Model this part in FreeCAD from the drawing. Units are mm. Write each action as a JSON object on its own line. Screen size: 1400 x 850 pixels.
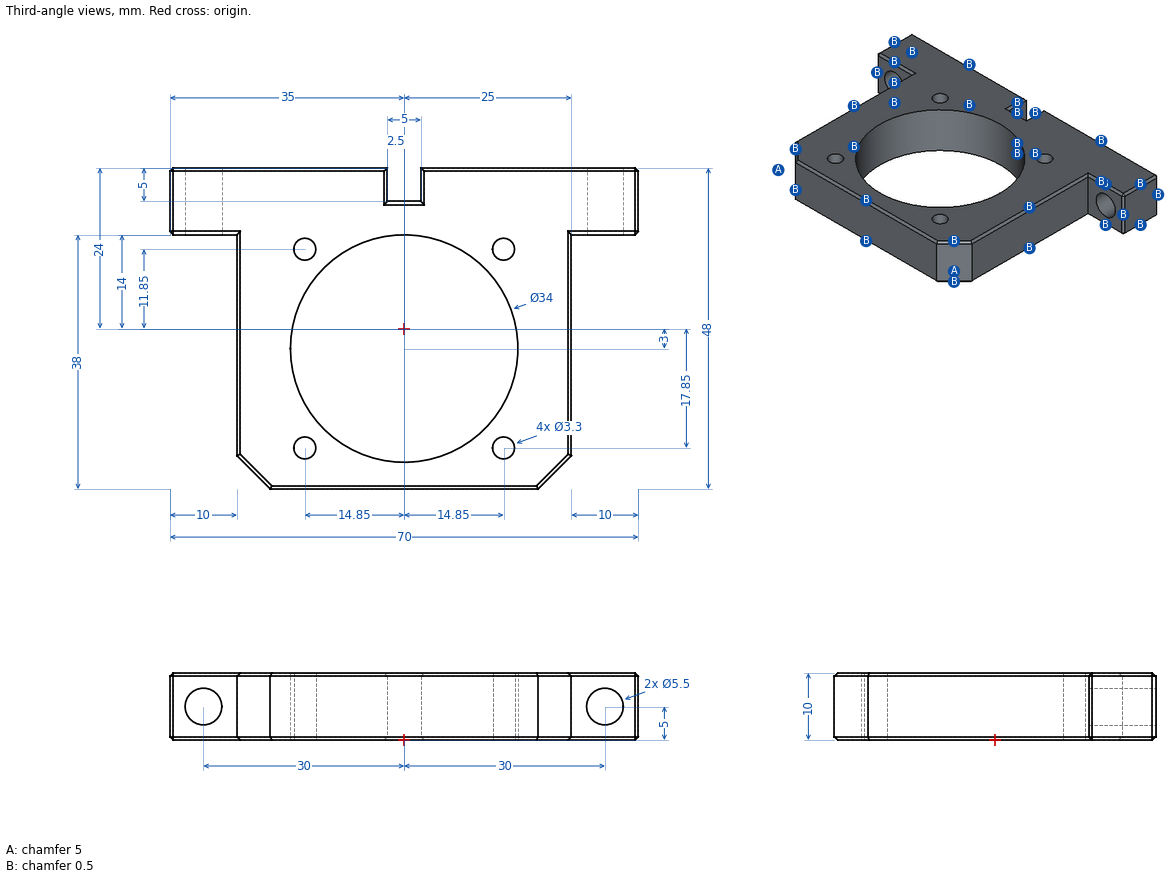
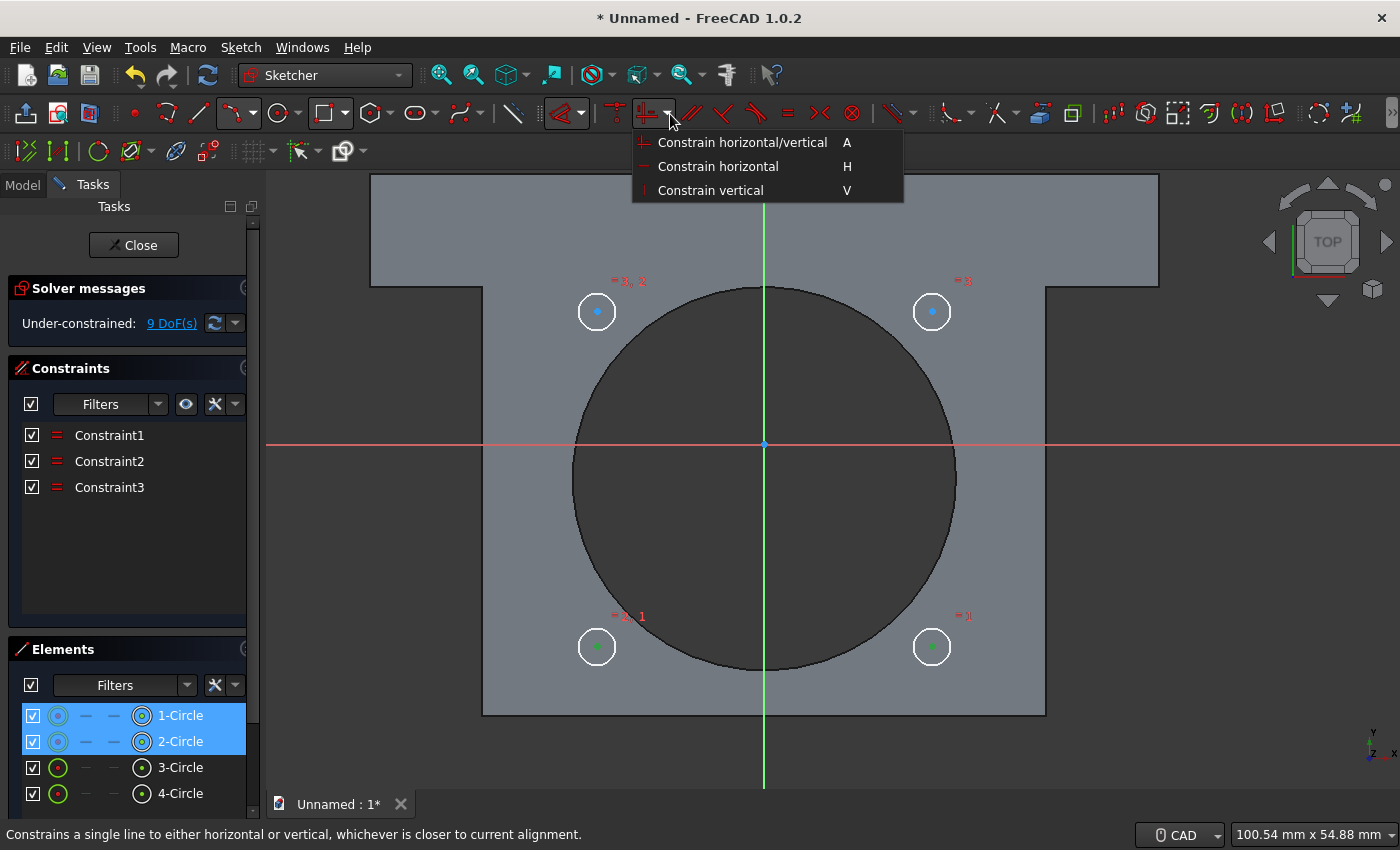
{"action": "left_click", "coordinate": [768, 166]}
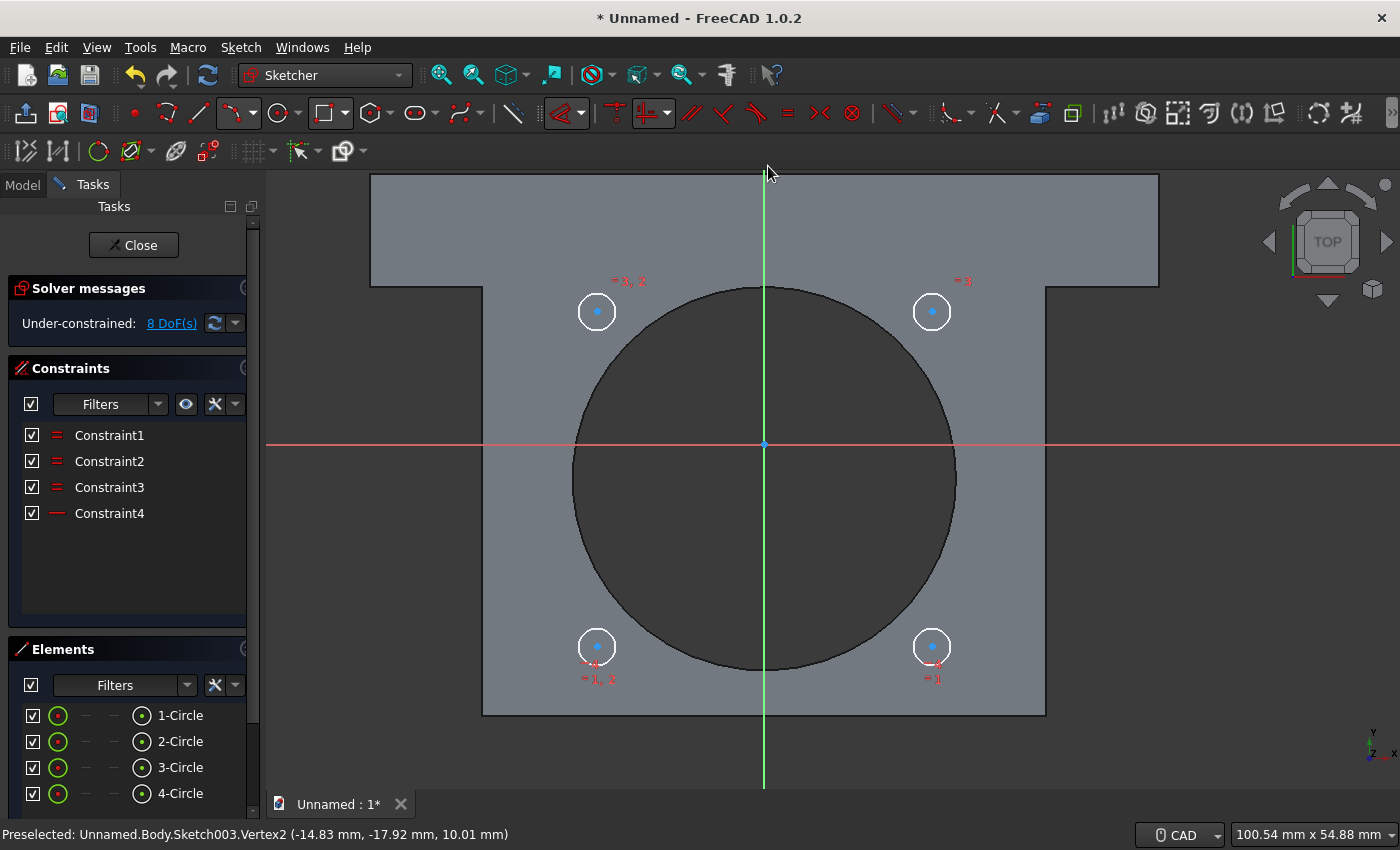
{"action": "left_click", "coordinate": [597, 647]}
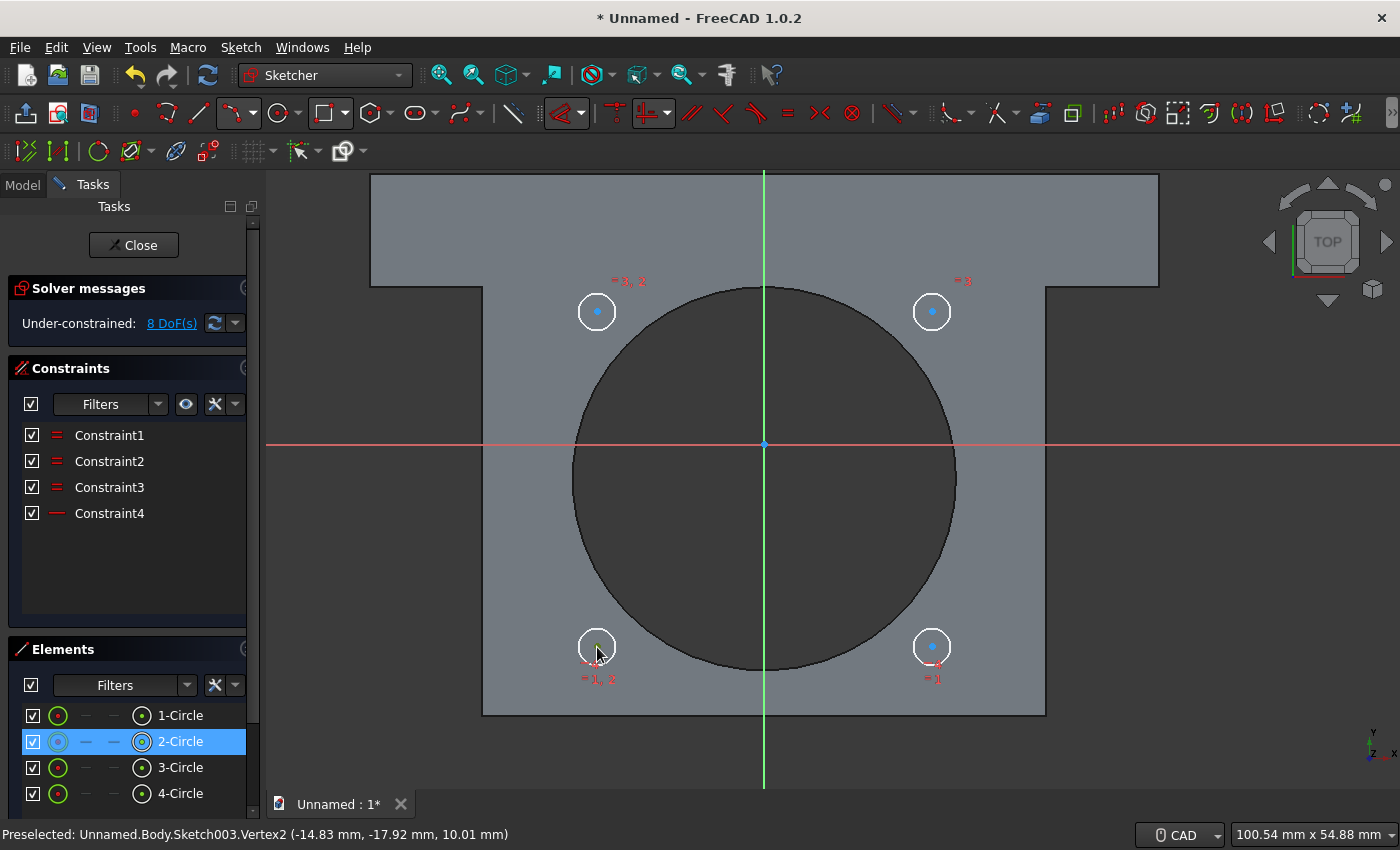
{"action": "left_click", "coordinate": [597, 312]}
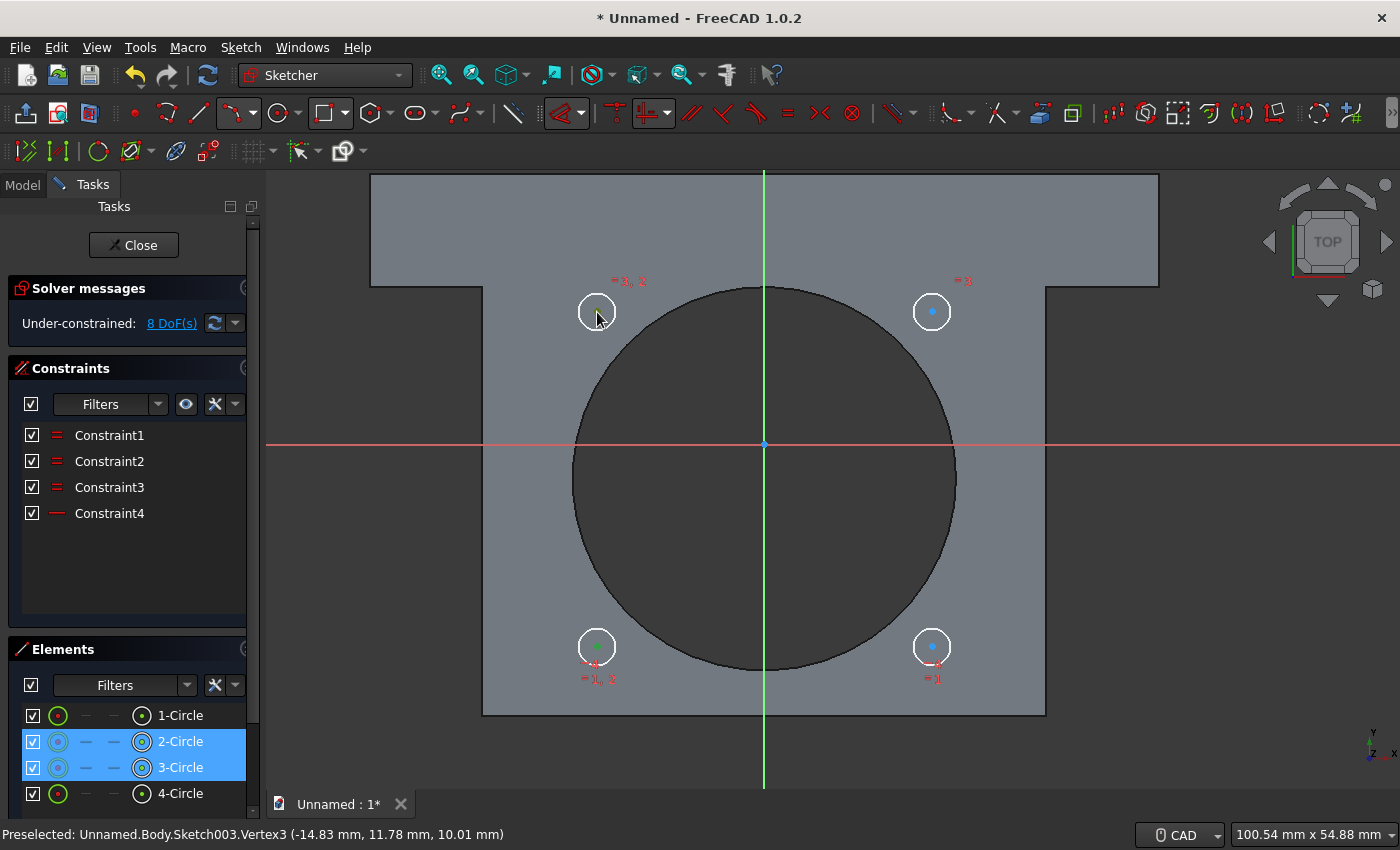
{"action": "key", "text": "v"}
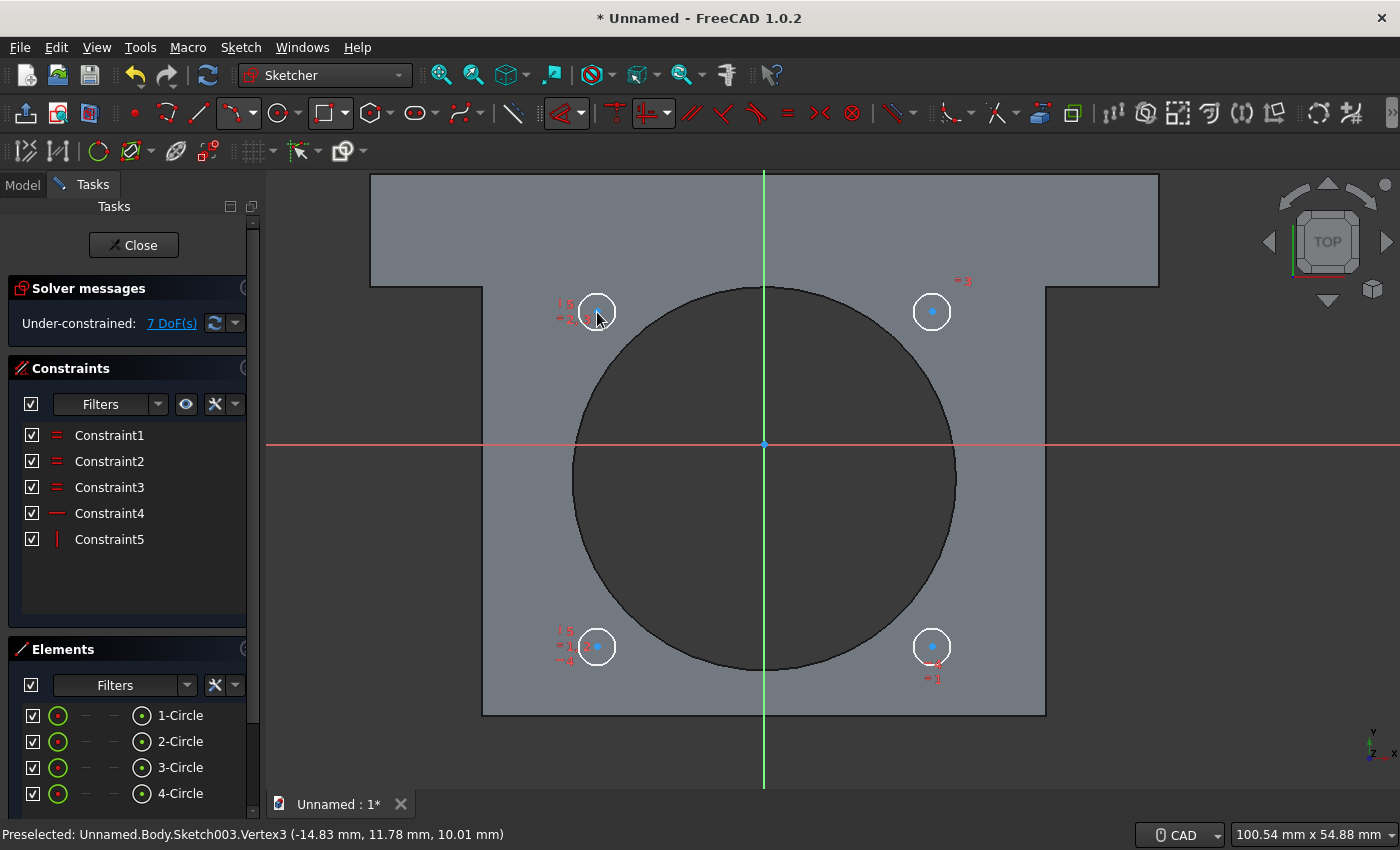
{"action": "left_click", "coordinate": [932, 647]}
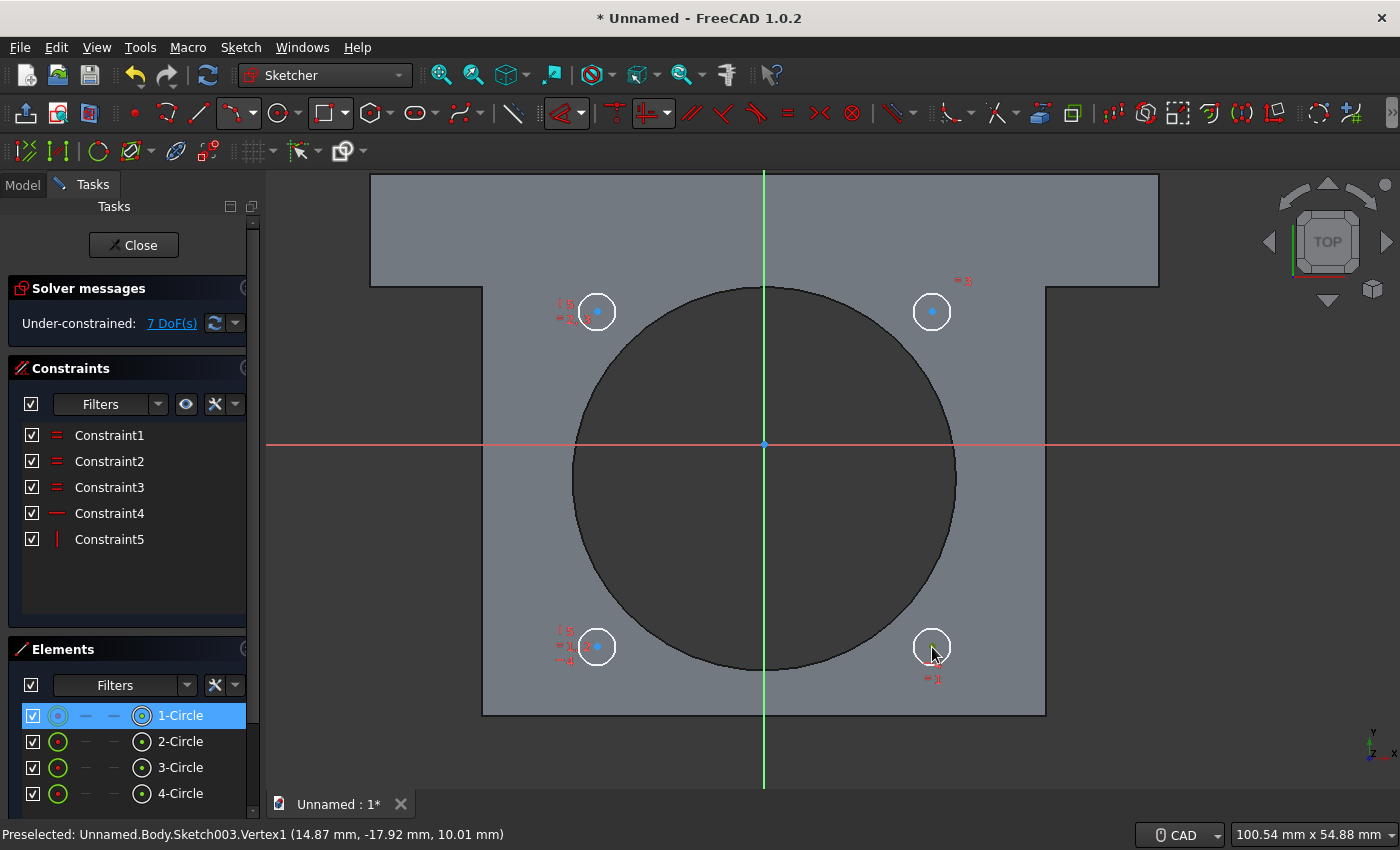
{"action": "left_click", "coordinate": [932, 312]}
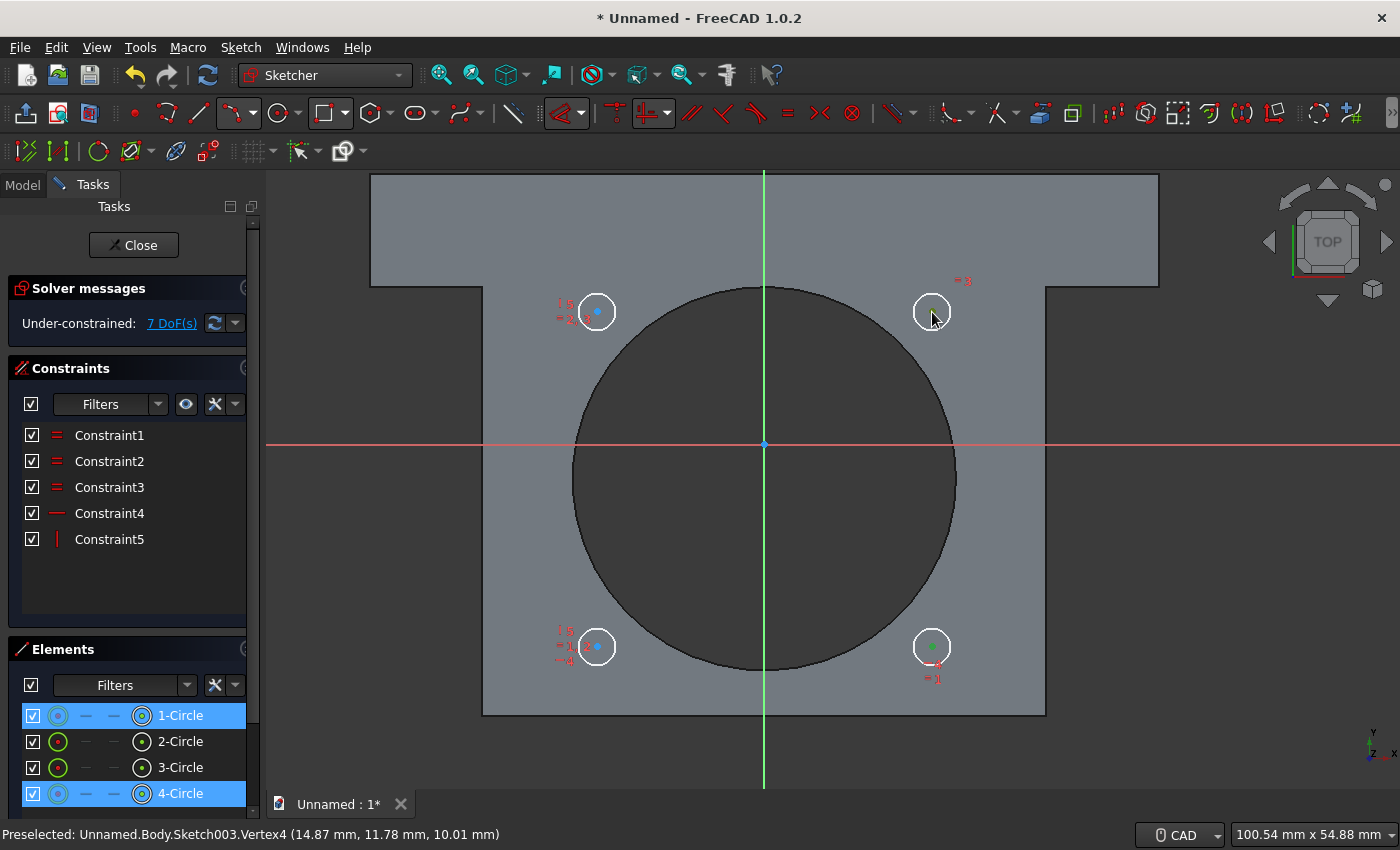
{"action": "left_click", "coordinate": [670, 114]}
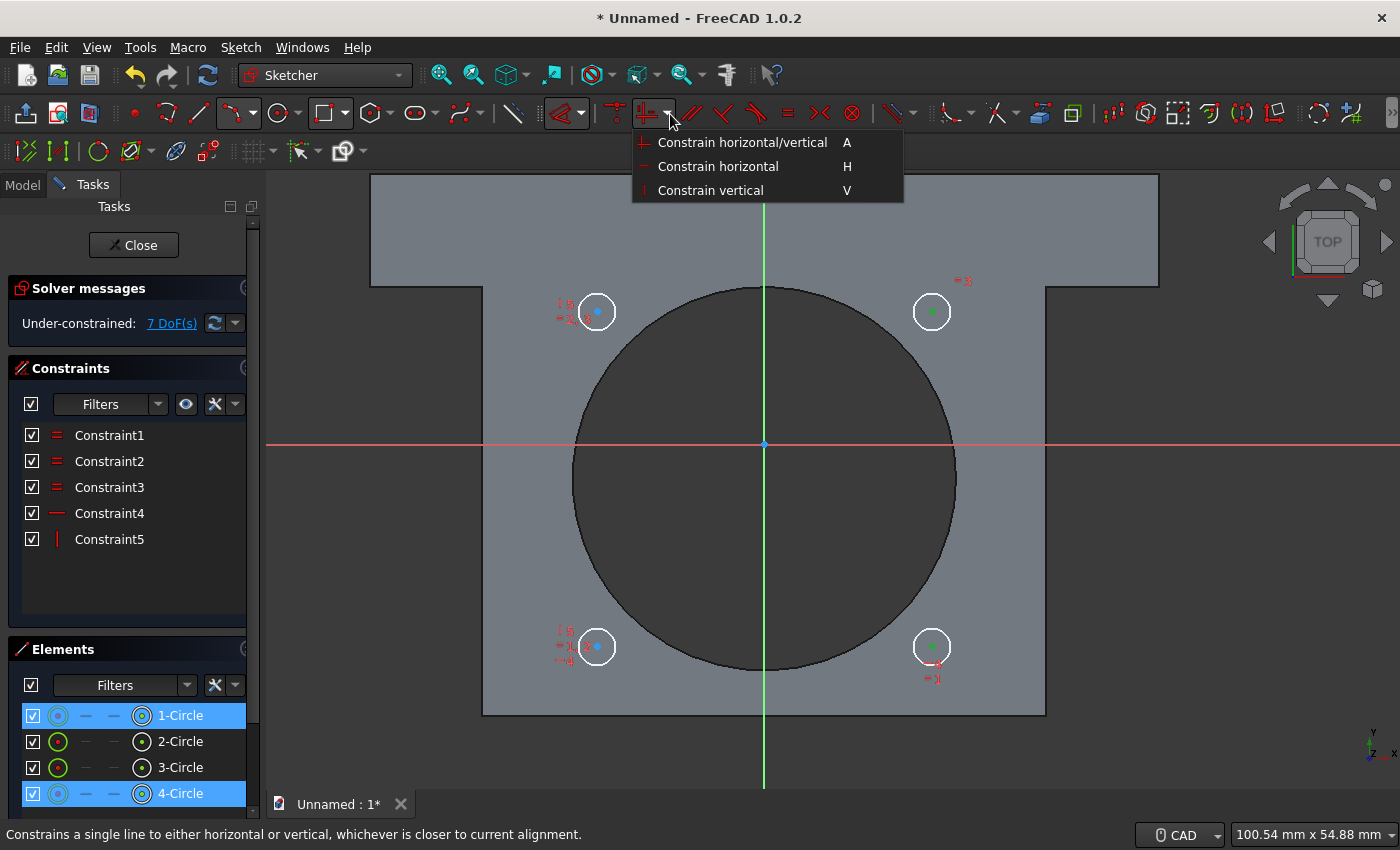
{"action": "left_click", "coordinate": [768, 190]}